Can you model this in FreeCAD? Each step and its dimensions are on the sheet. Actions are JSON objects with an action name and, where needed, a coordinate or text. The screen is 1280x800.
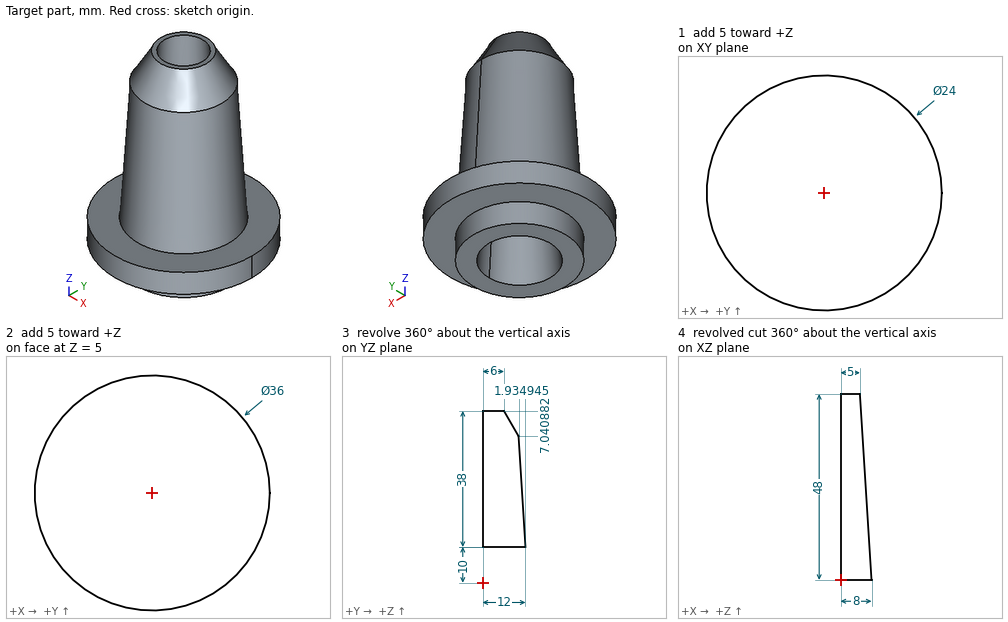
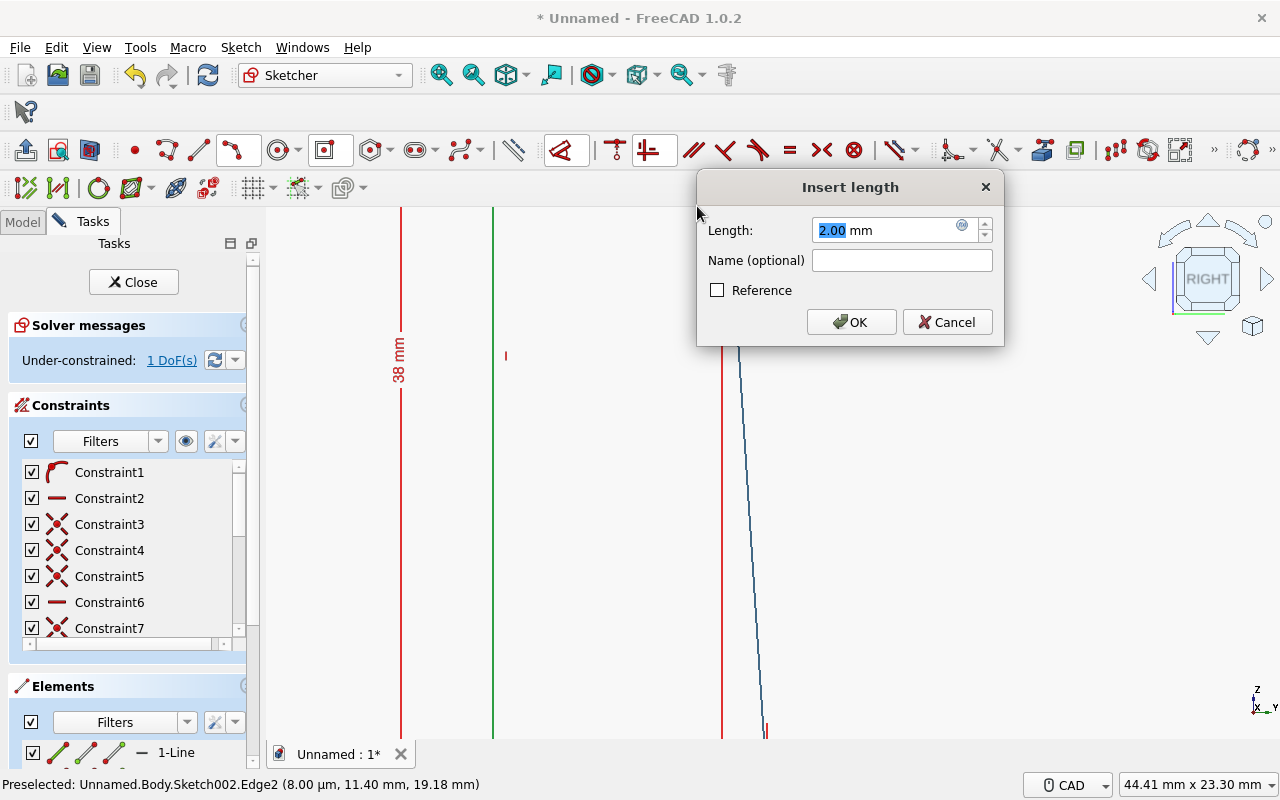
{"action": "type", "text": "1.934945"}
{"action": "key", "text": "Return"}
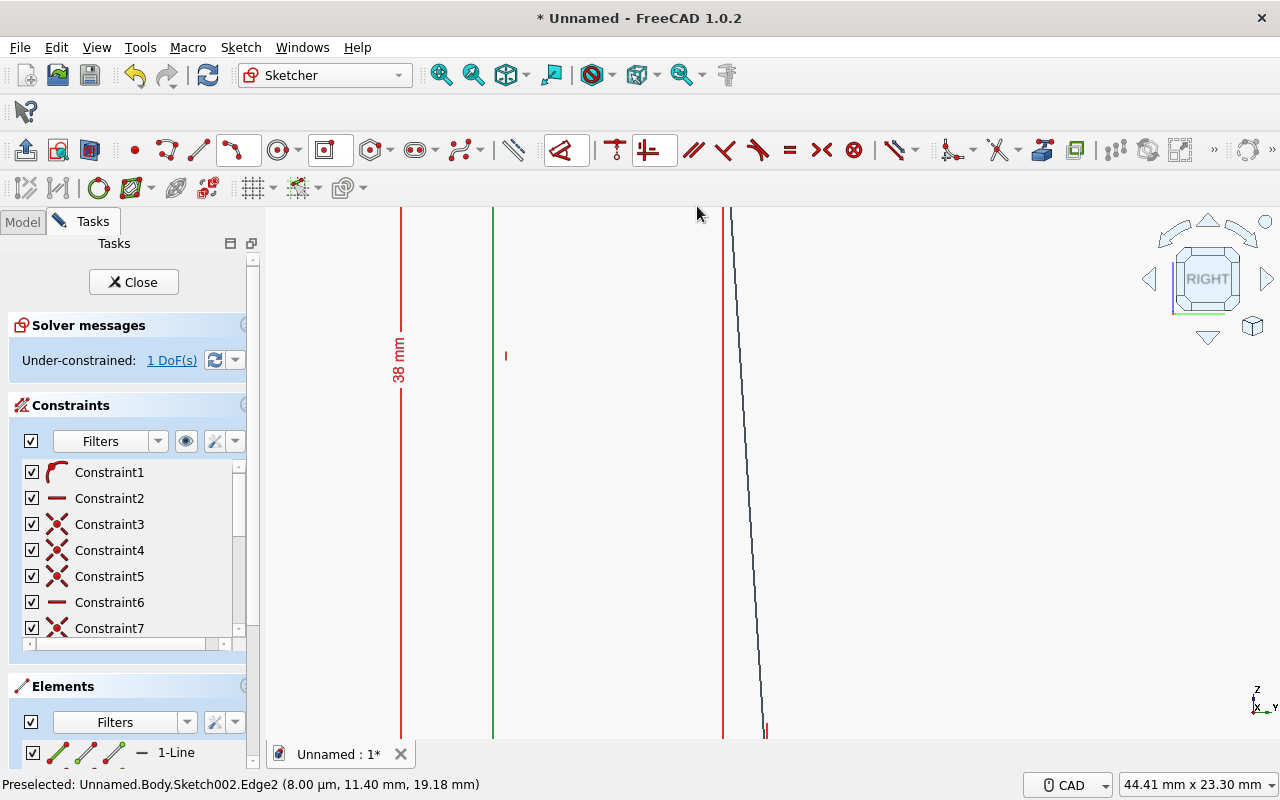
{"action": "scroll", "coordinate": [736, 474], "scroll_direction": "down", "scroll_amount": 6}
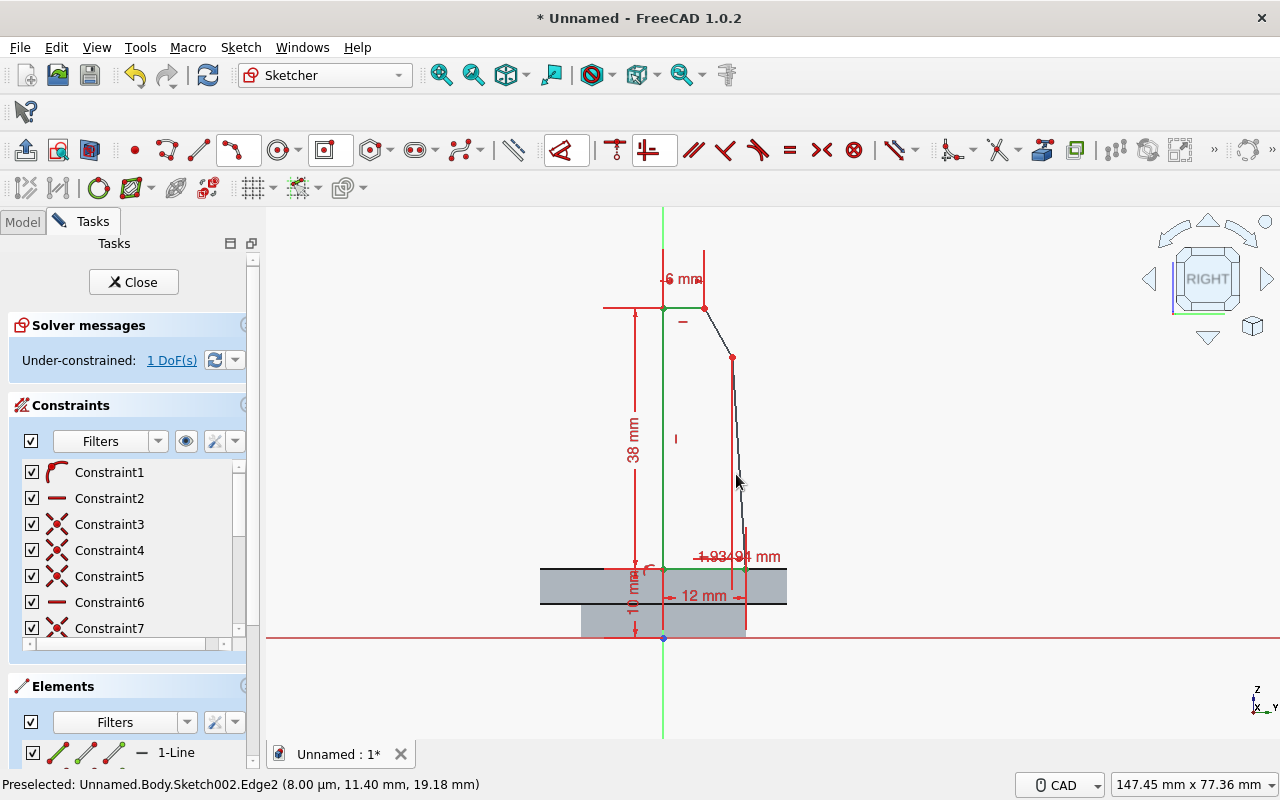
{"action": "left_click", "coordinate": [724, 343]}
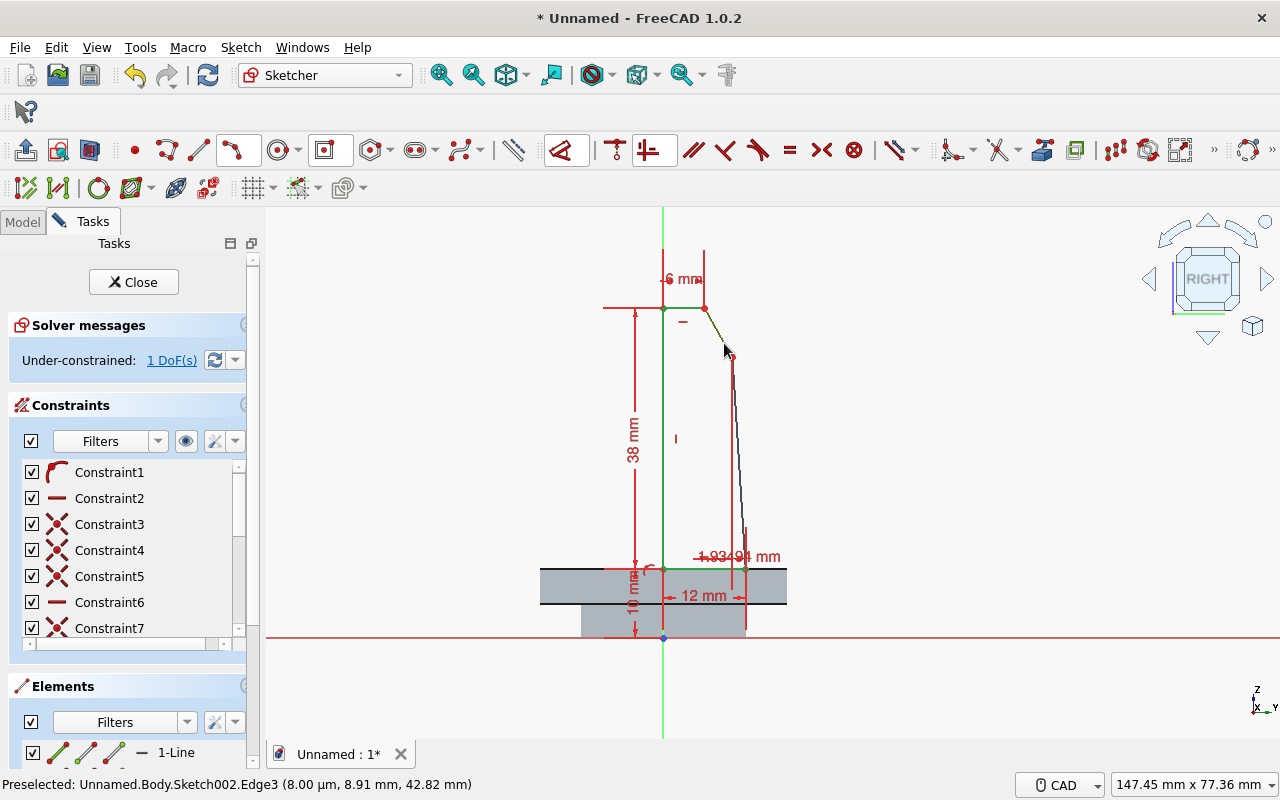
{"action": "key", "text": "i"}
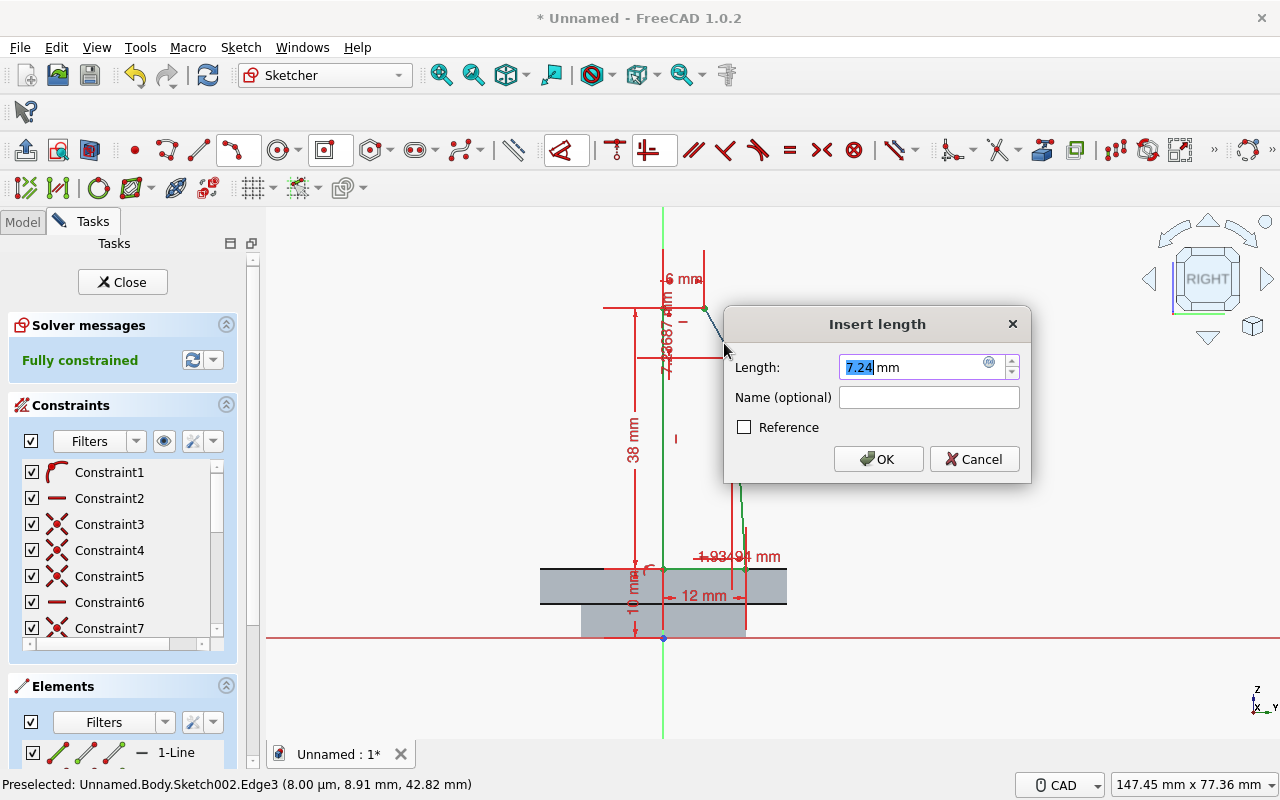
{"action": "type", "text": "7.040882"}
{"action": "key", "text": "Return"}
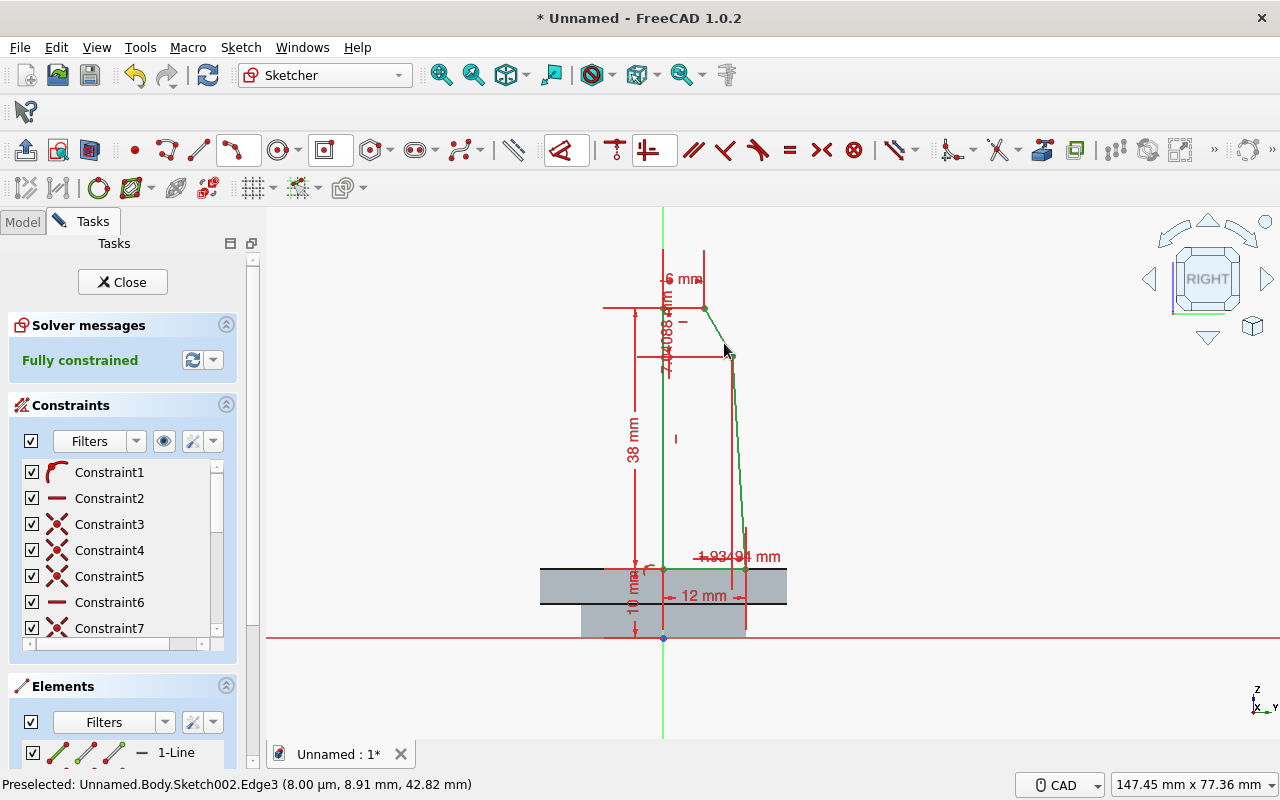
{"action": "left_click", "coordinate": [123, 282]}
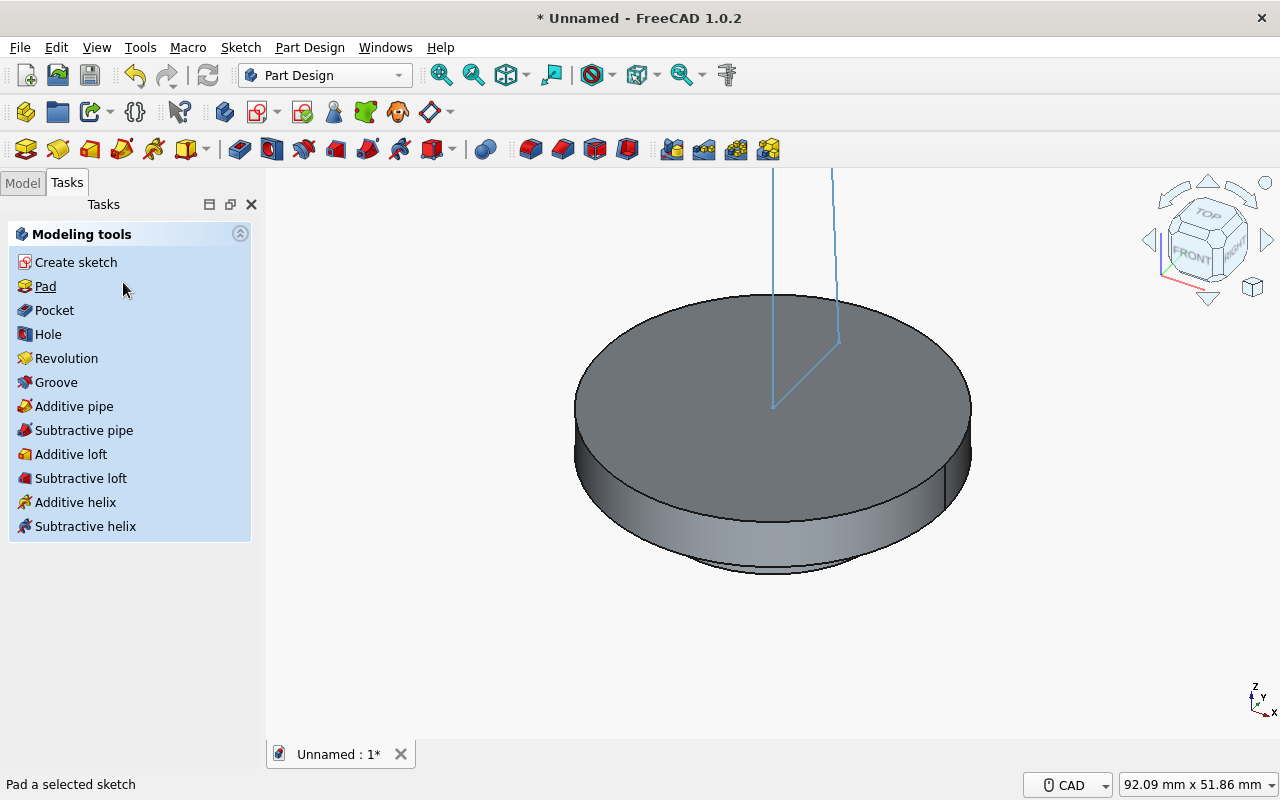
{"action": "left_click", "coordinate": [58, 150]}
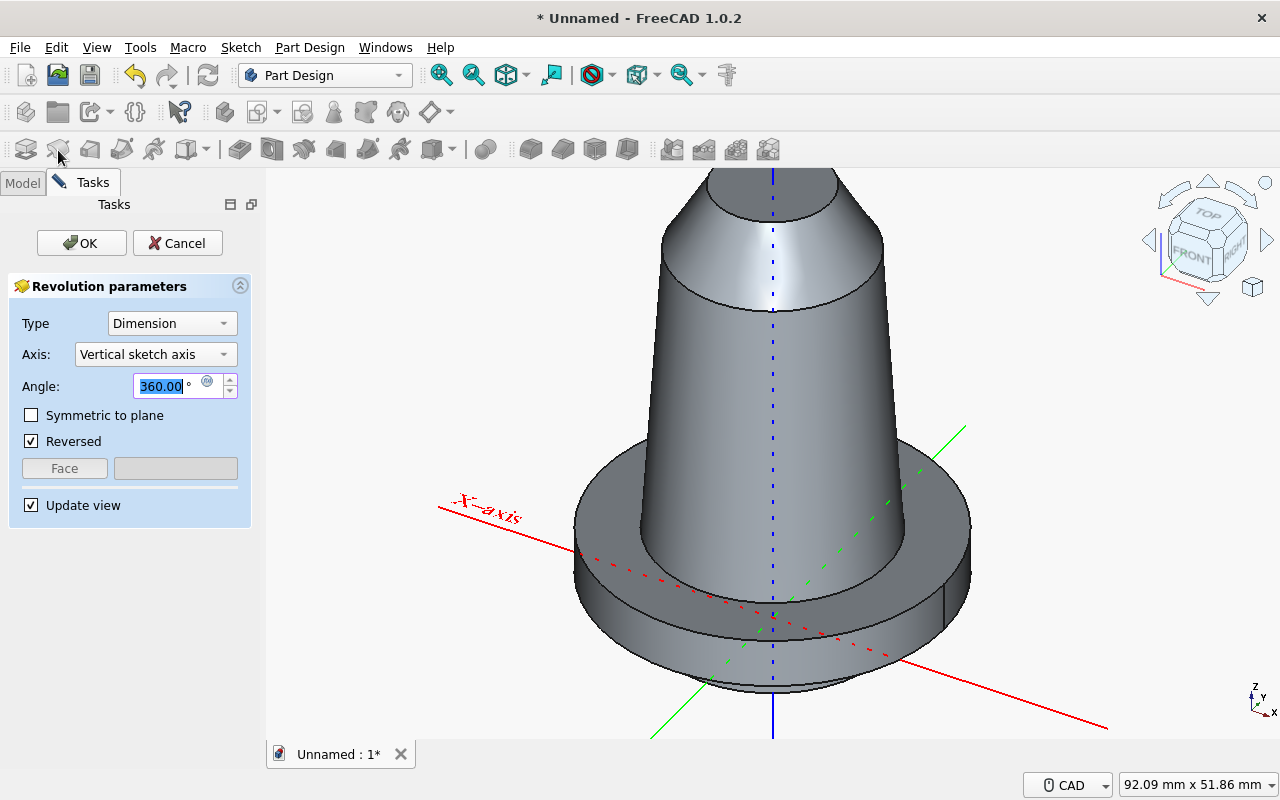
{"action": "left_click", "coordinate": [82, 243]}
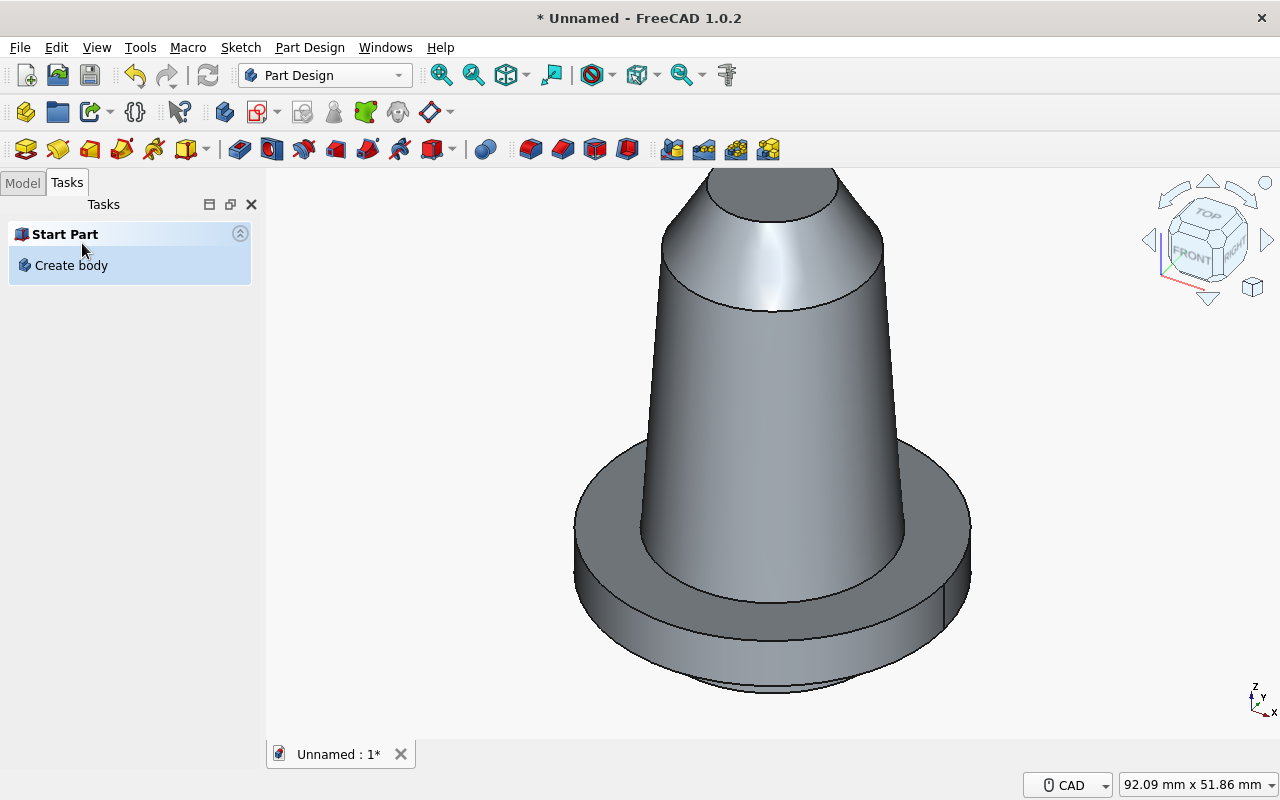
{"action": "left_click", "coordinate": [442, 76]}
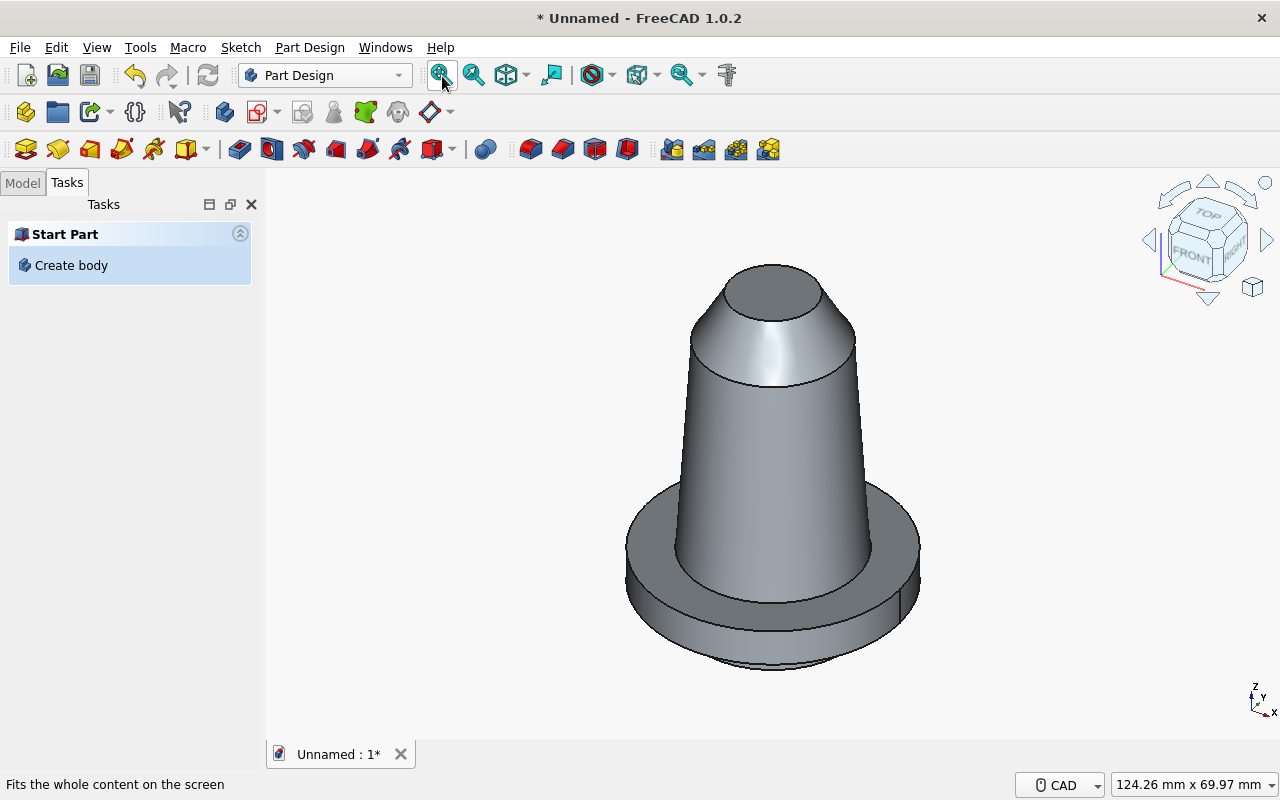
{"action": "left_click", "coordinate": [258, 112]}